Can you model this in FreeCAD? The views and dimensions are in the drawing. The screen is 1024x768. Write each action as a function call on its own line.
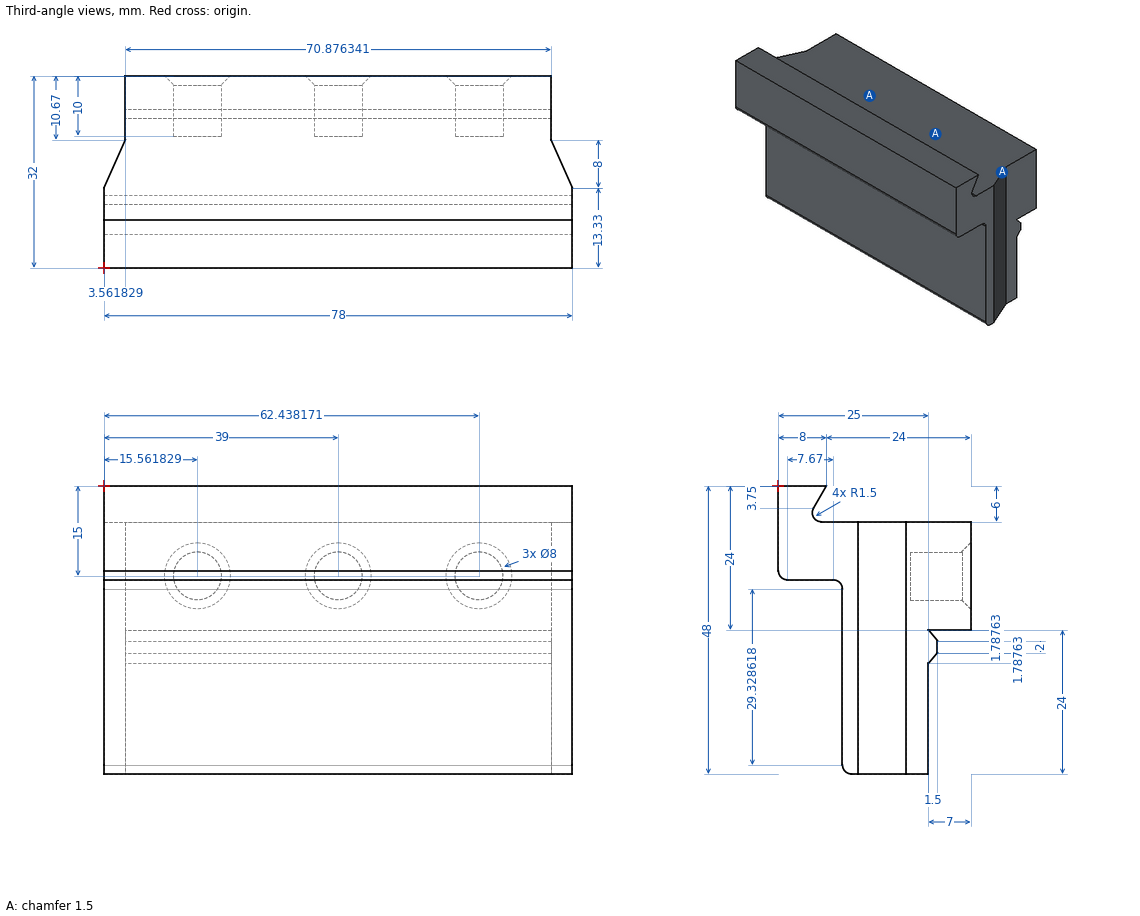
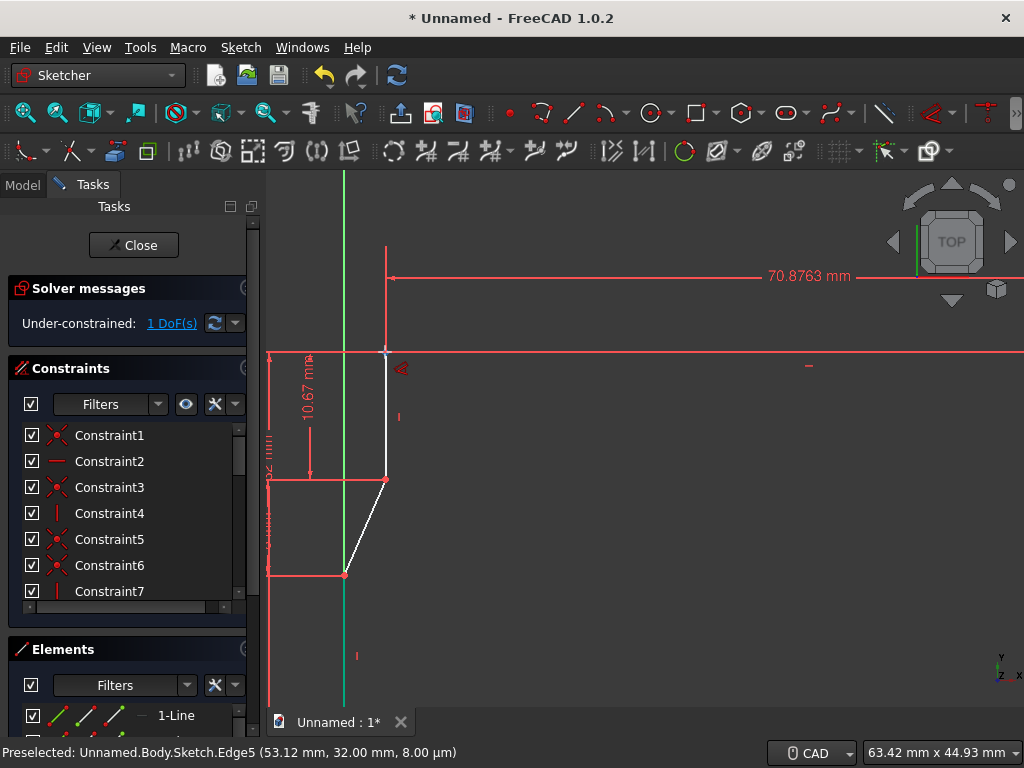
click(386, 352)
click(365, 318)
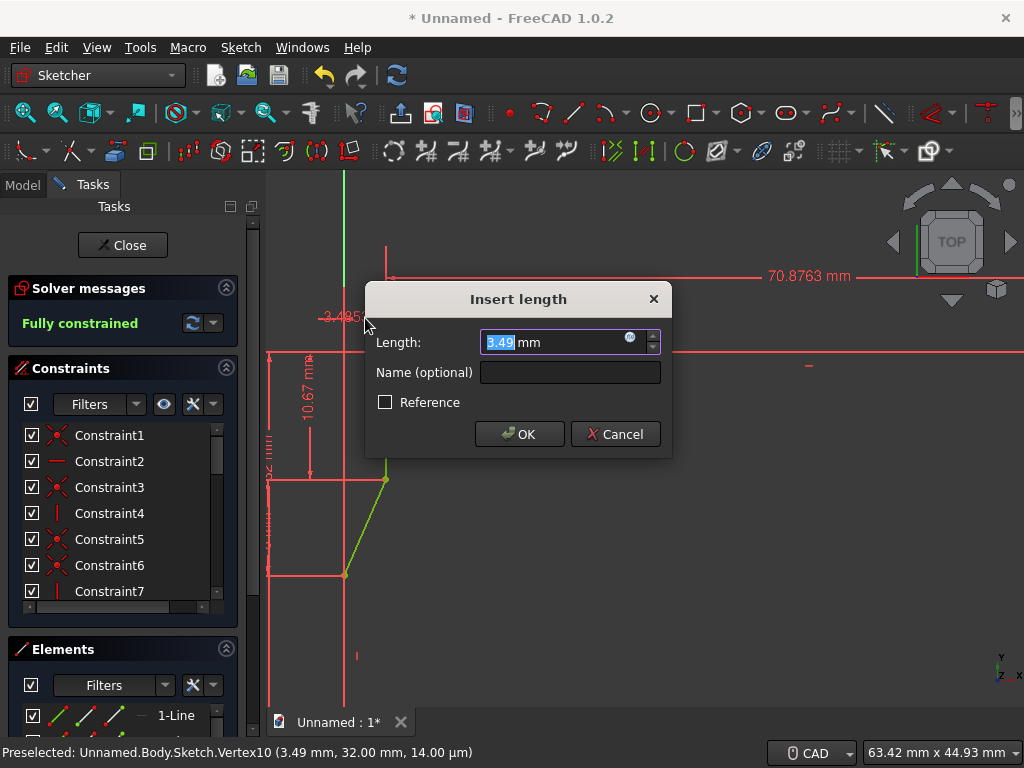
text(3.561829)
key(Return)
key(Escape)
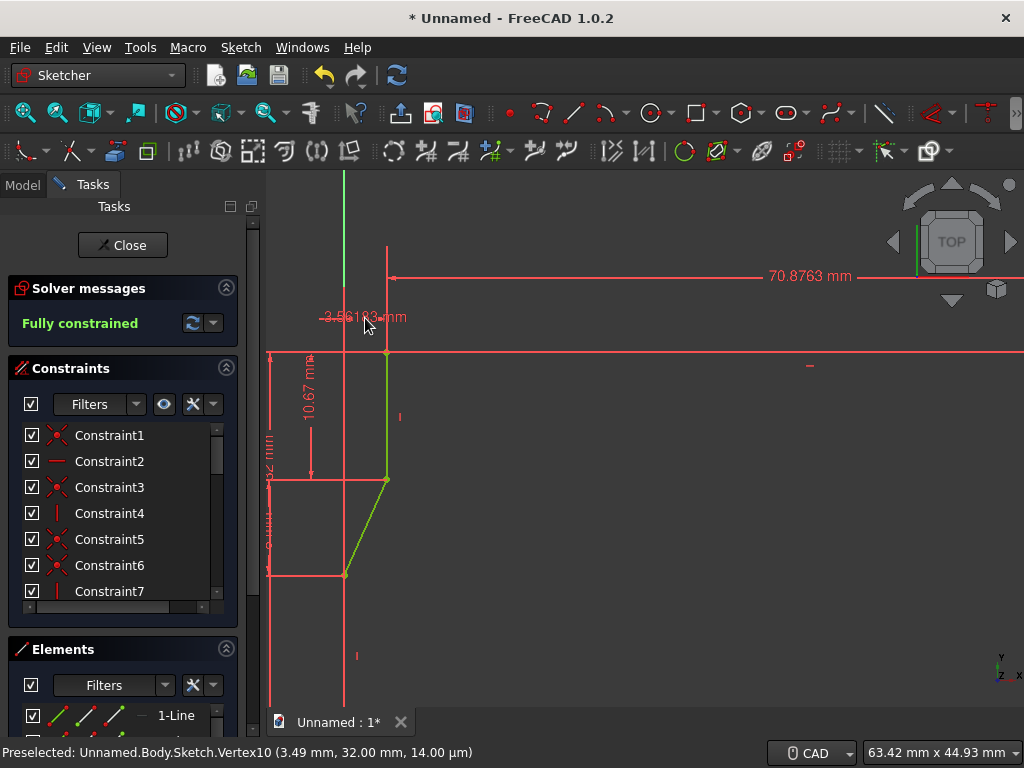
click(123, 245)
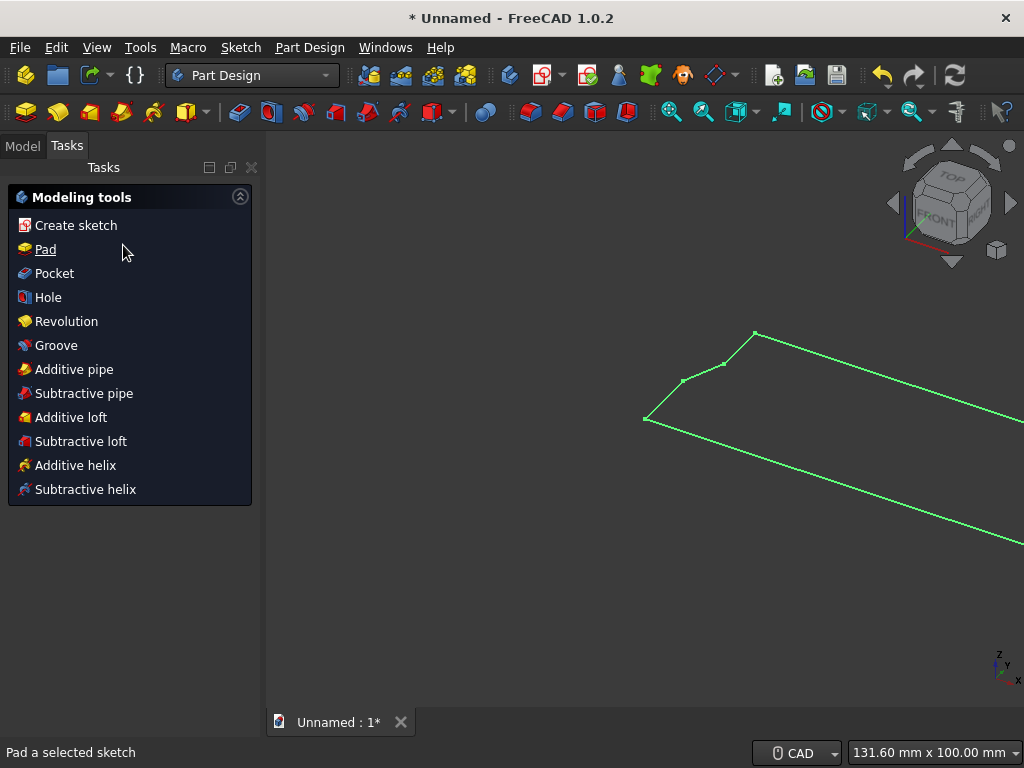
click(26, 112)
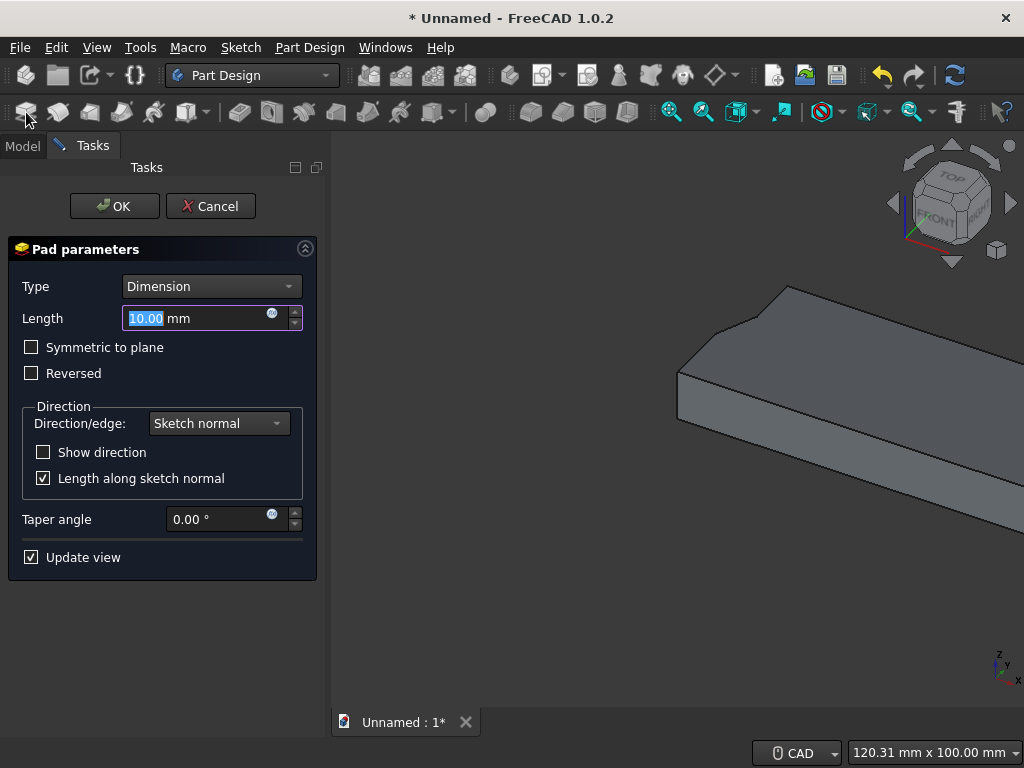
text(48)
key(Tab)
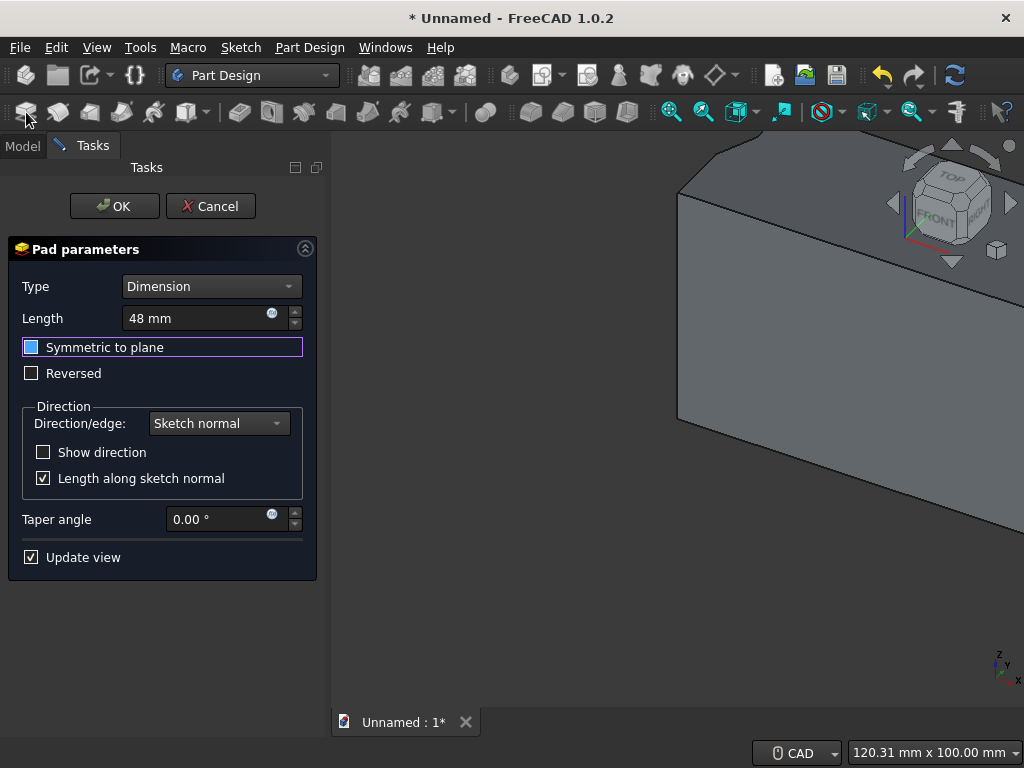
click(30, 373)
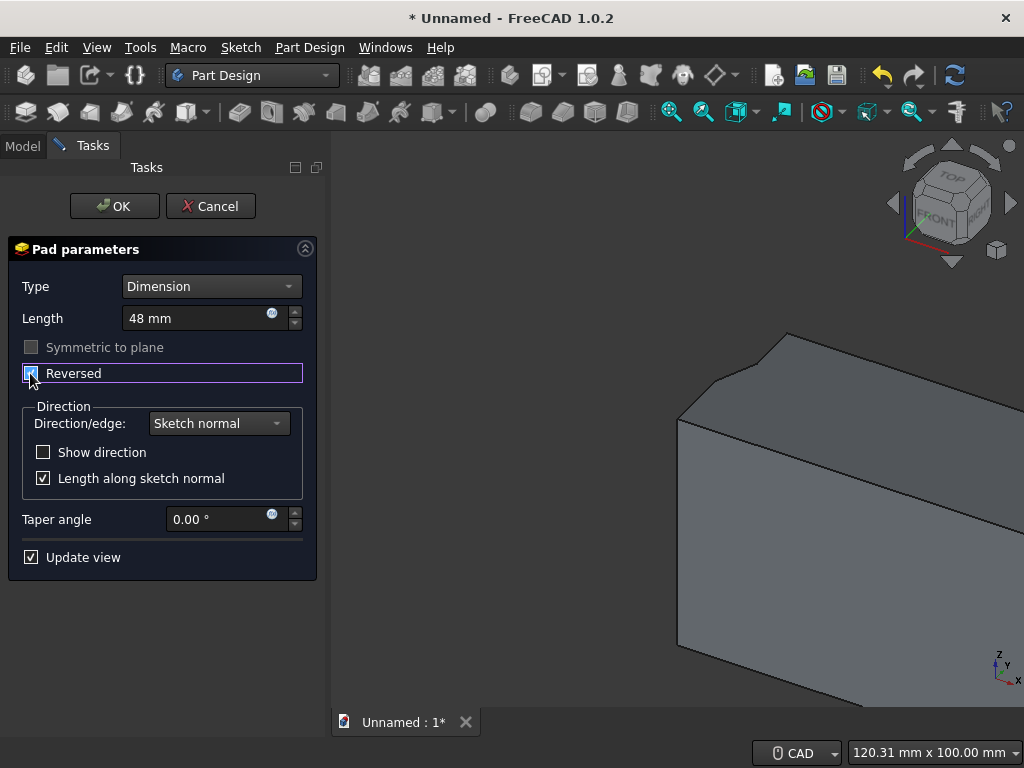
click(115, 206)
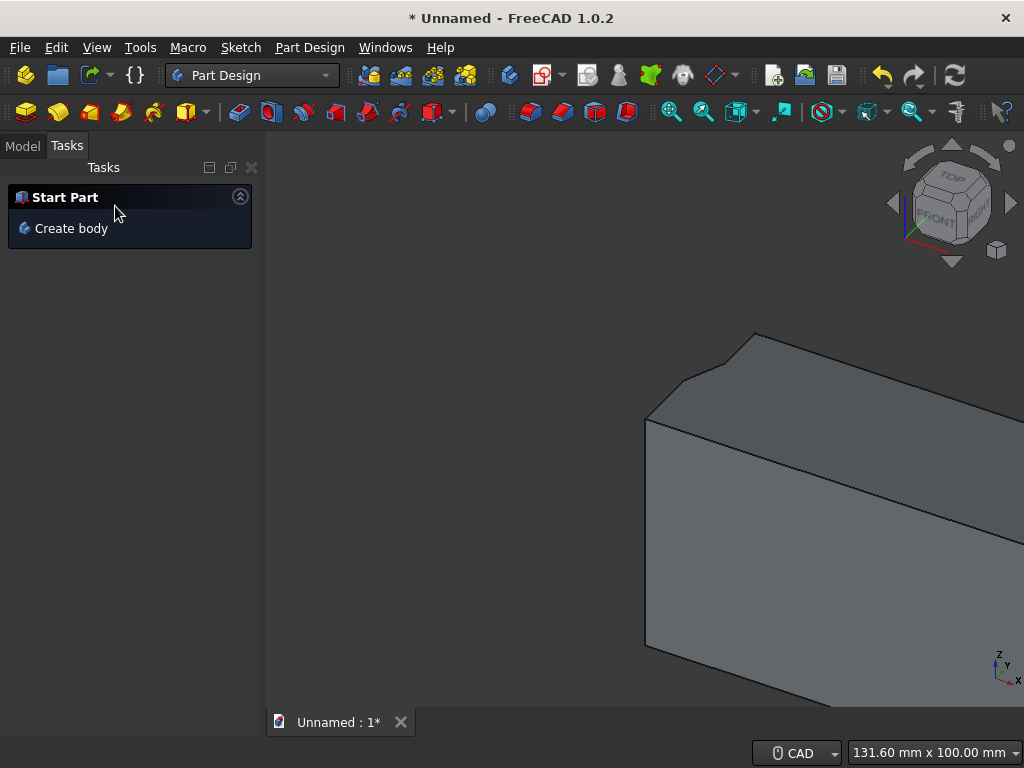
click(672, 112)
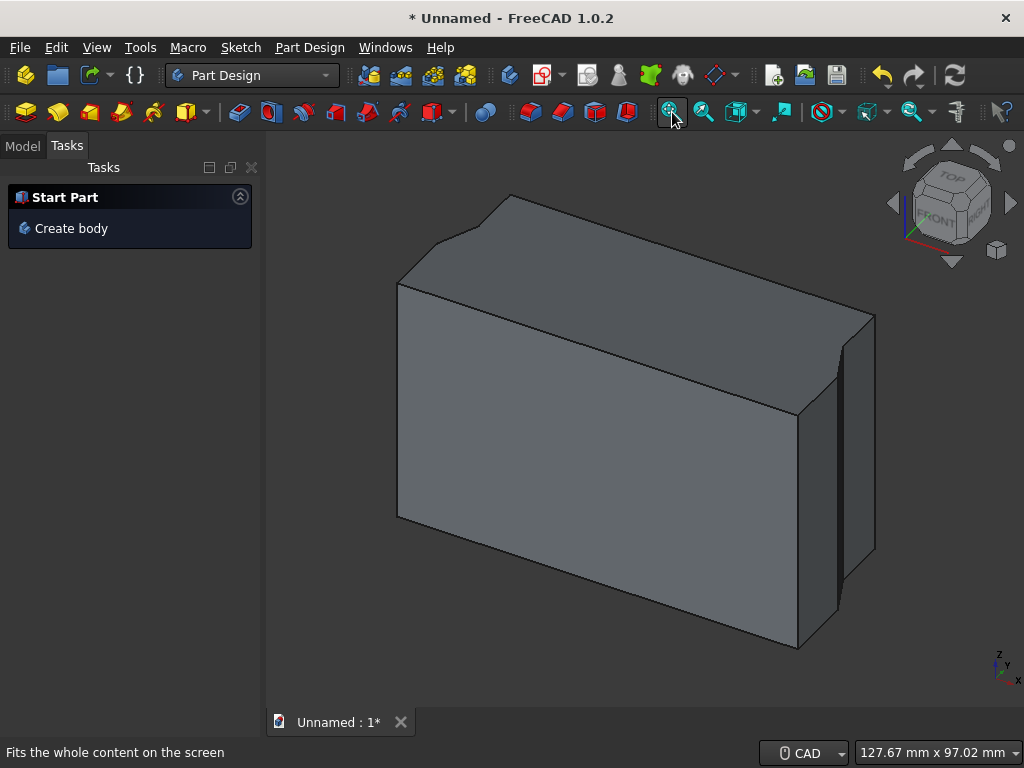
click(818, 445)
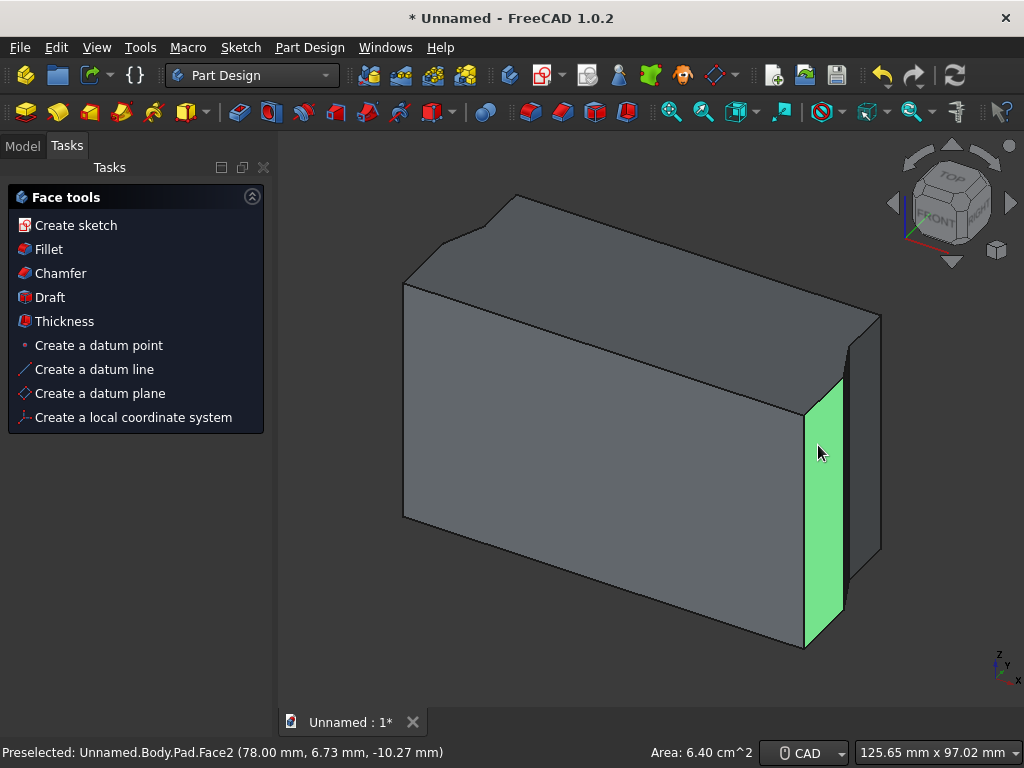
click(542, 76)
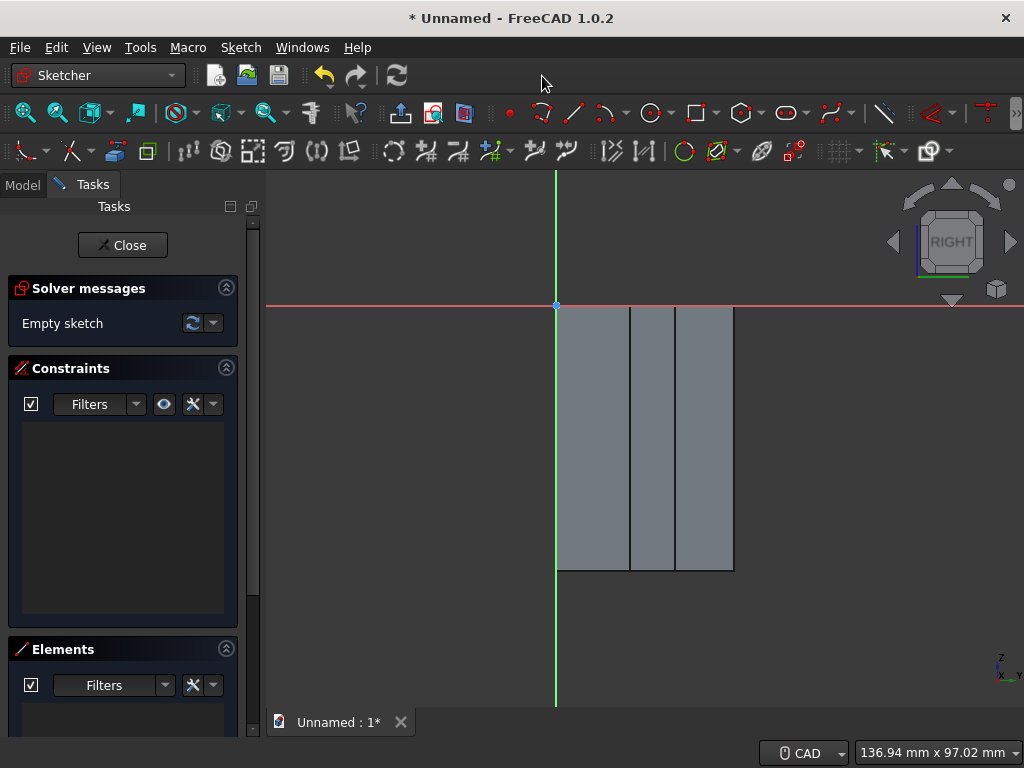
click(542, 114)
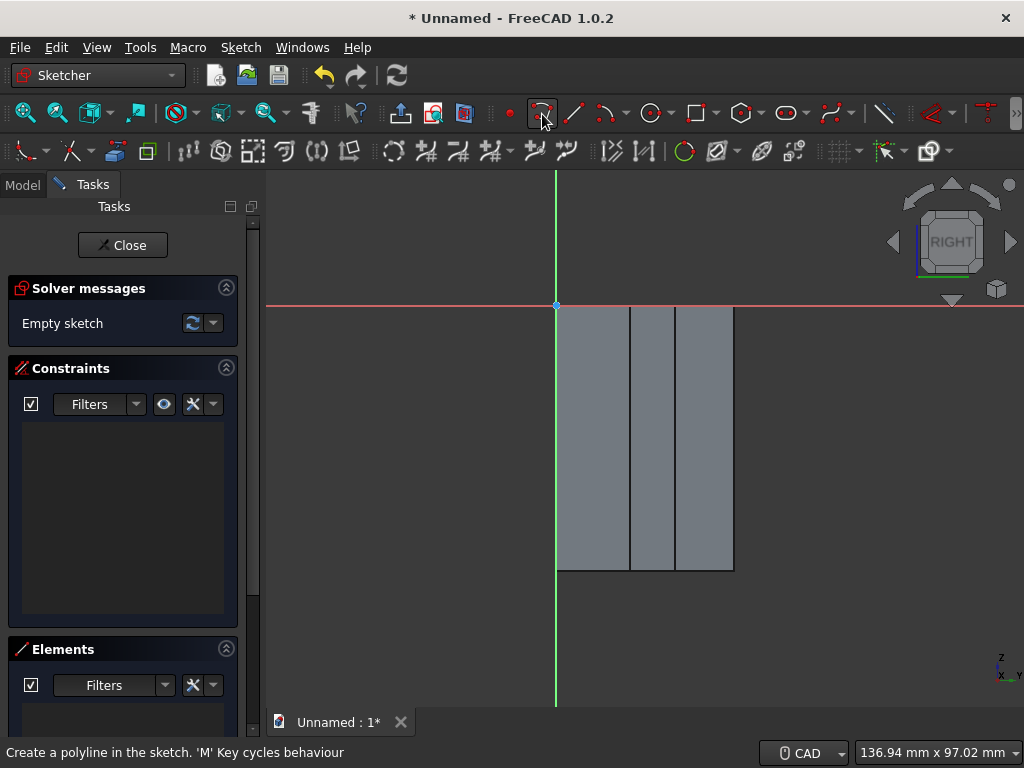
click(596, 339)
click(734, 339)
click(734, 306)
click(601, 315)
click(589, 326)
right_click(589, 326)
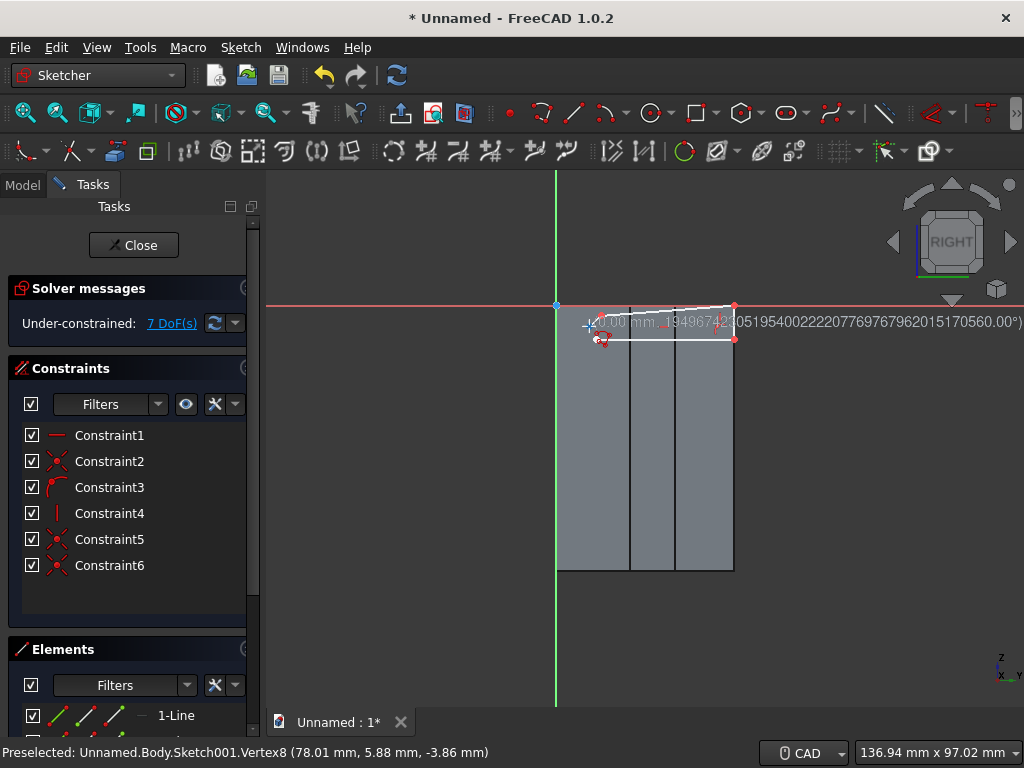
click(628, 114)